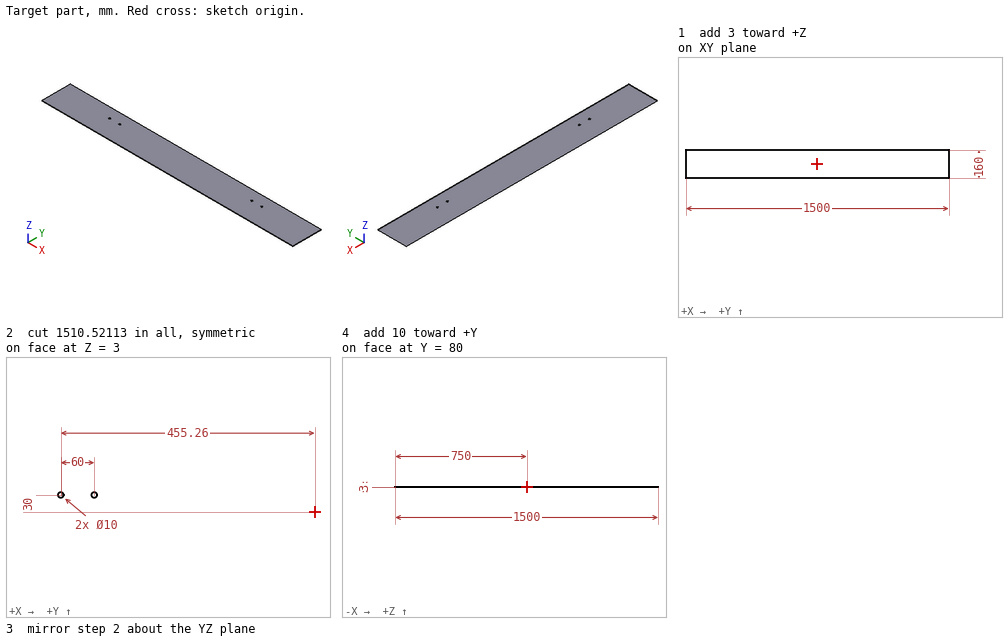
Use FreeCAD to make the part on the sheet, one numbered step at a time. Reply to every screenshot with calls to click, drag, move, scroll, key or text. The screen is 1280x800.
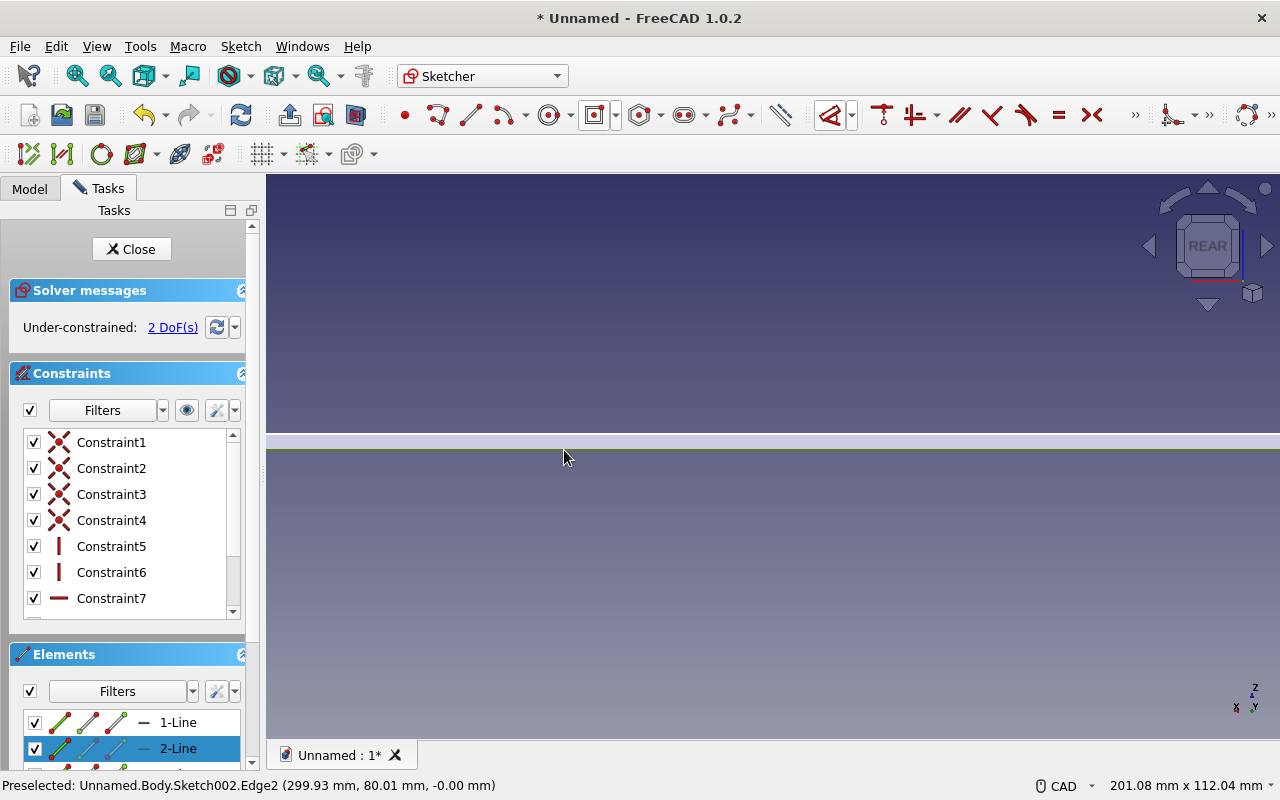
key(l)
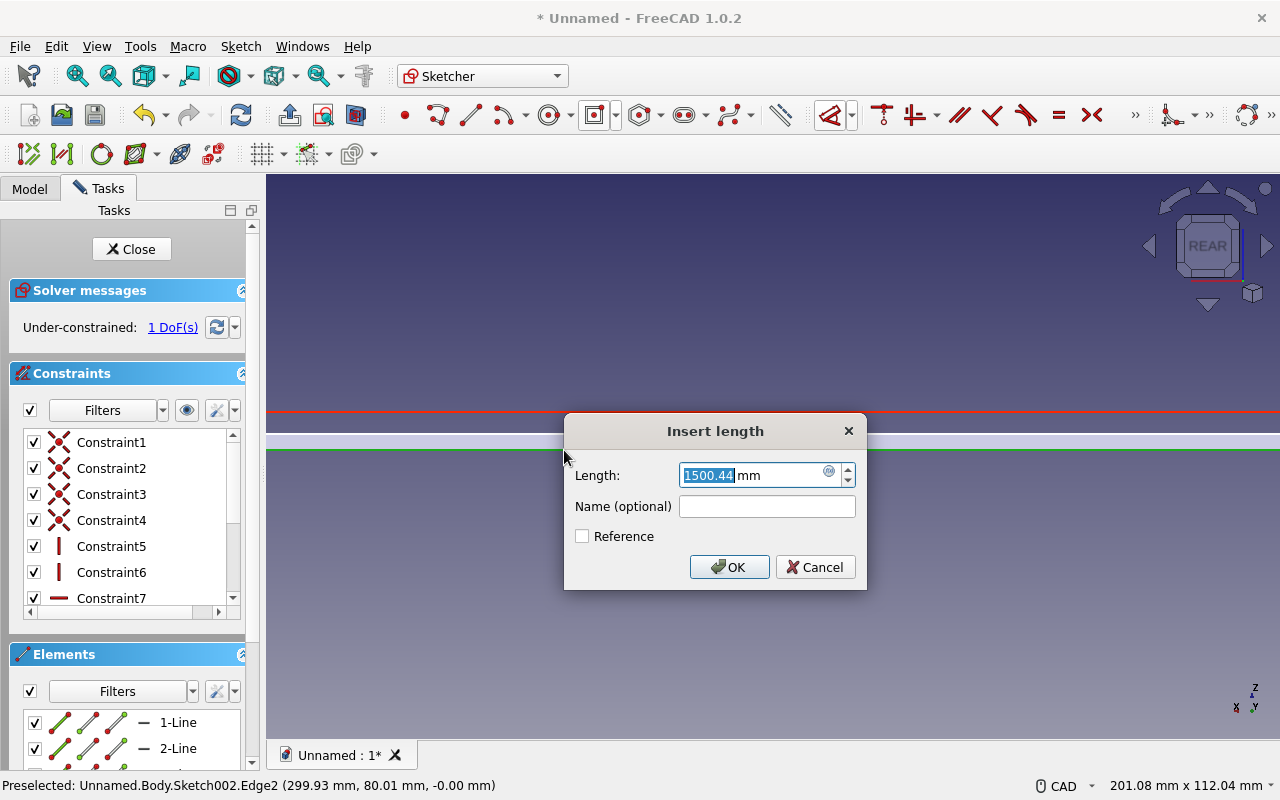
text(1500)
key(Return)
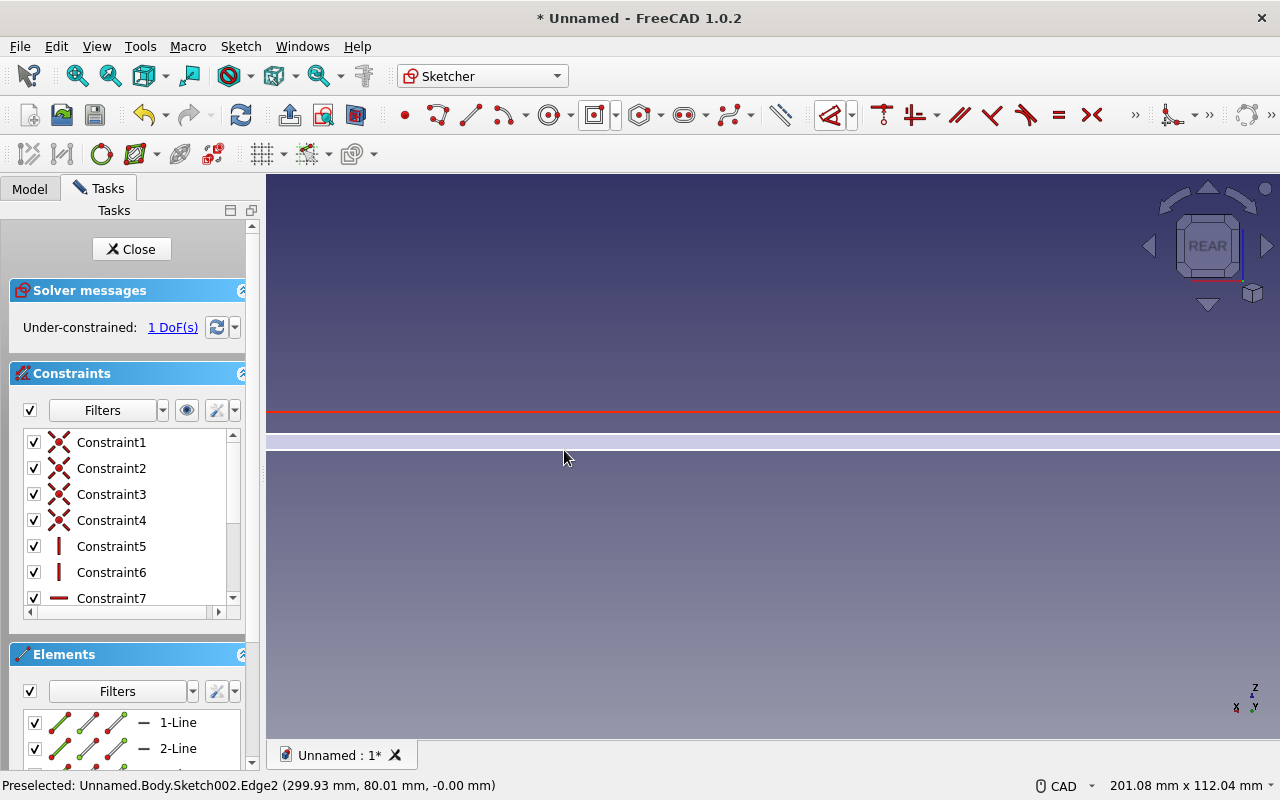
scroll(594, 458, down, 13)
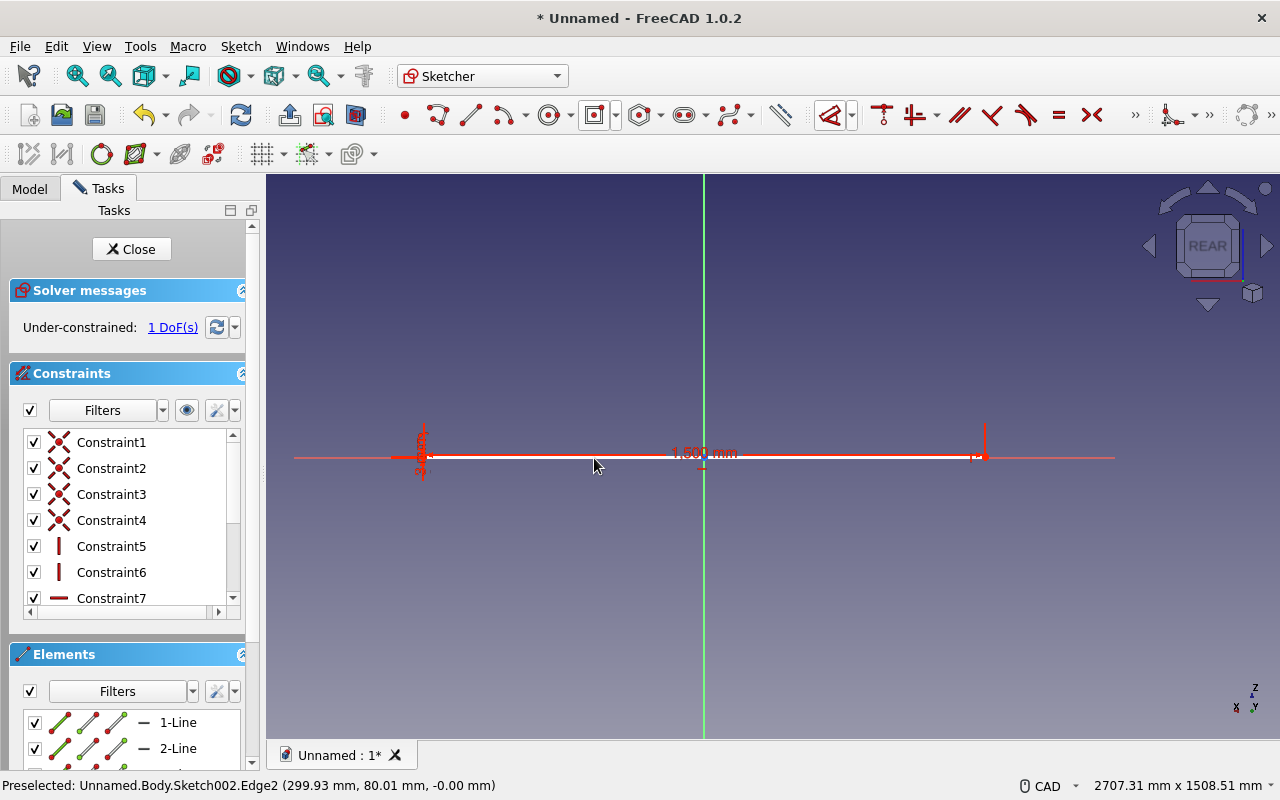
scroll(424, 457, up, 12)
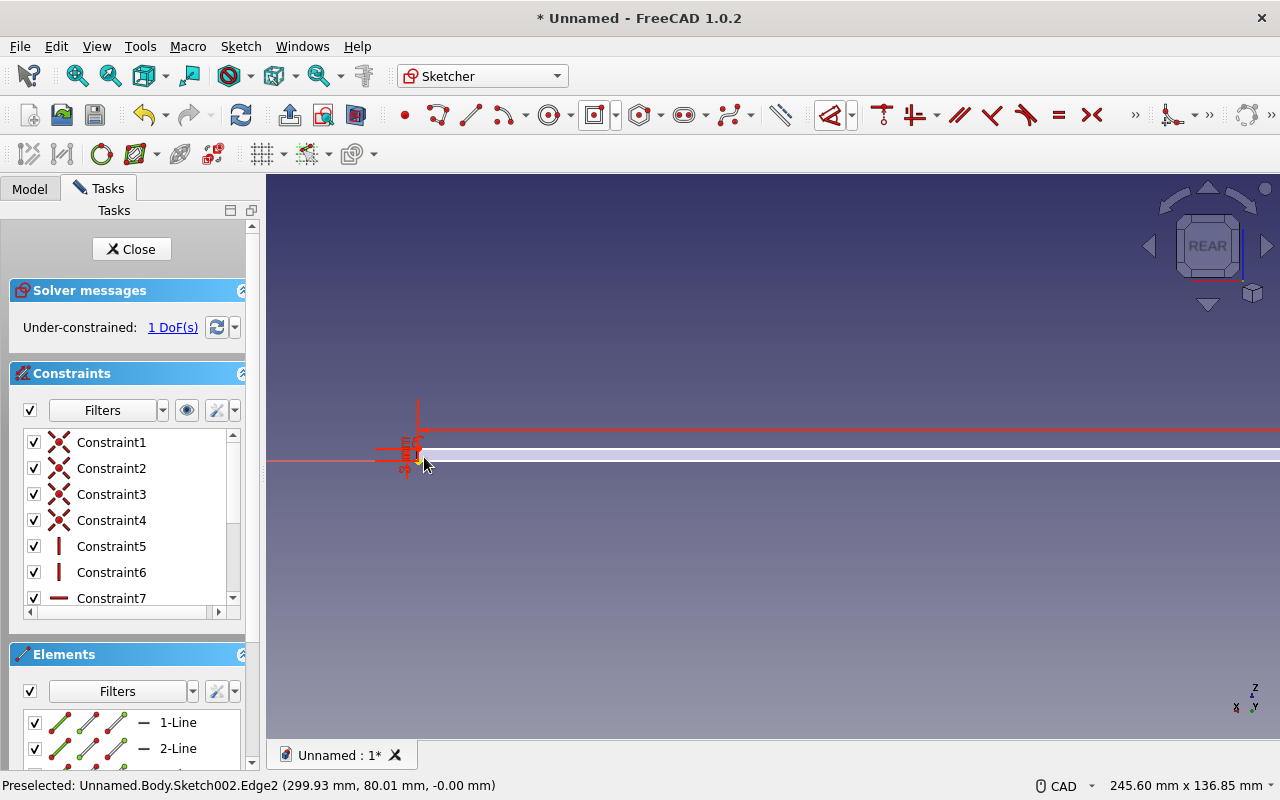
click(418, 449)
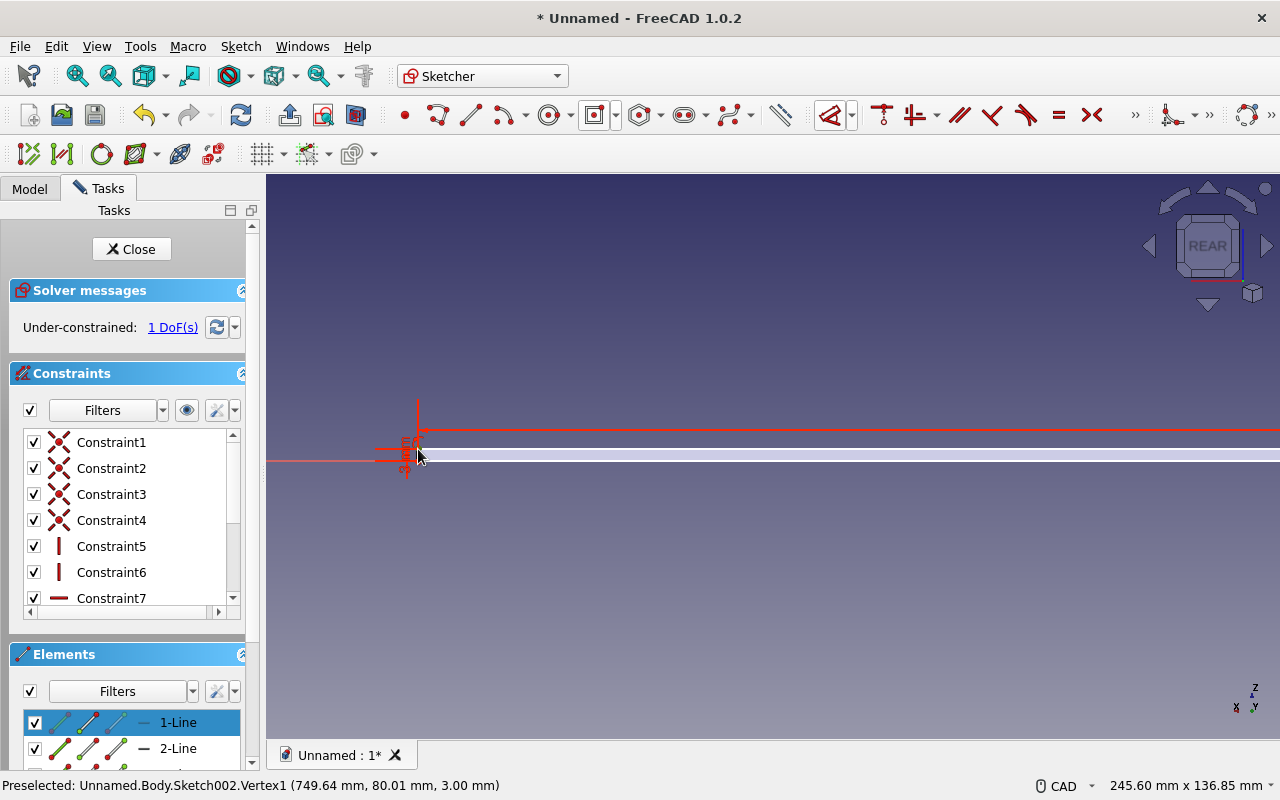
click(852, 116)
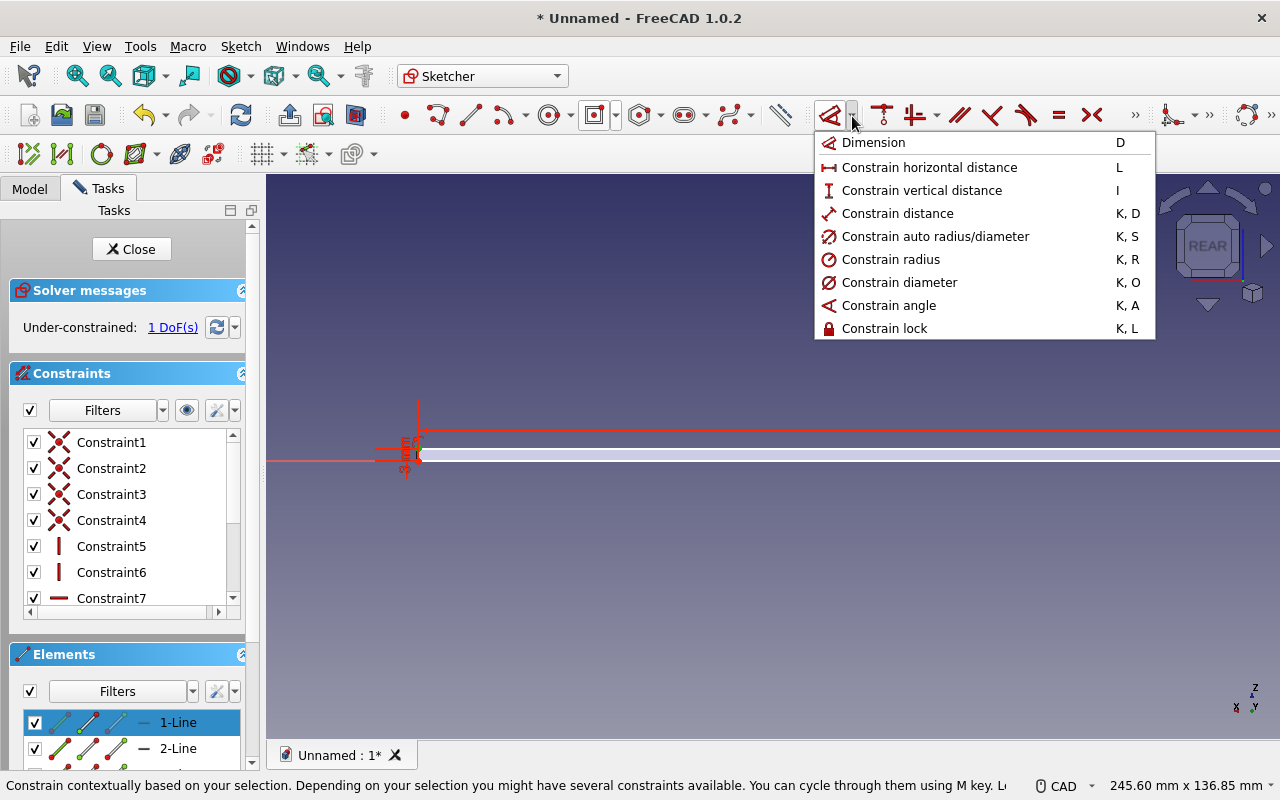
click(985, 168)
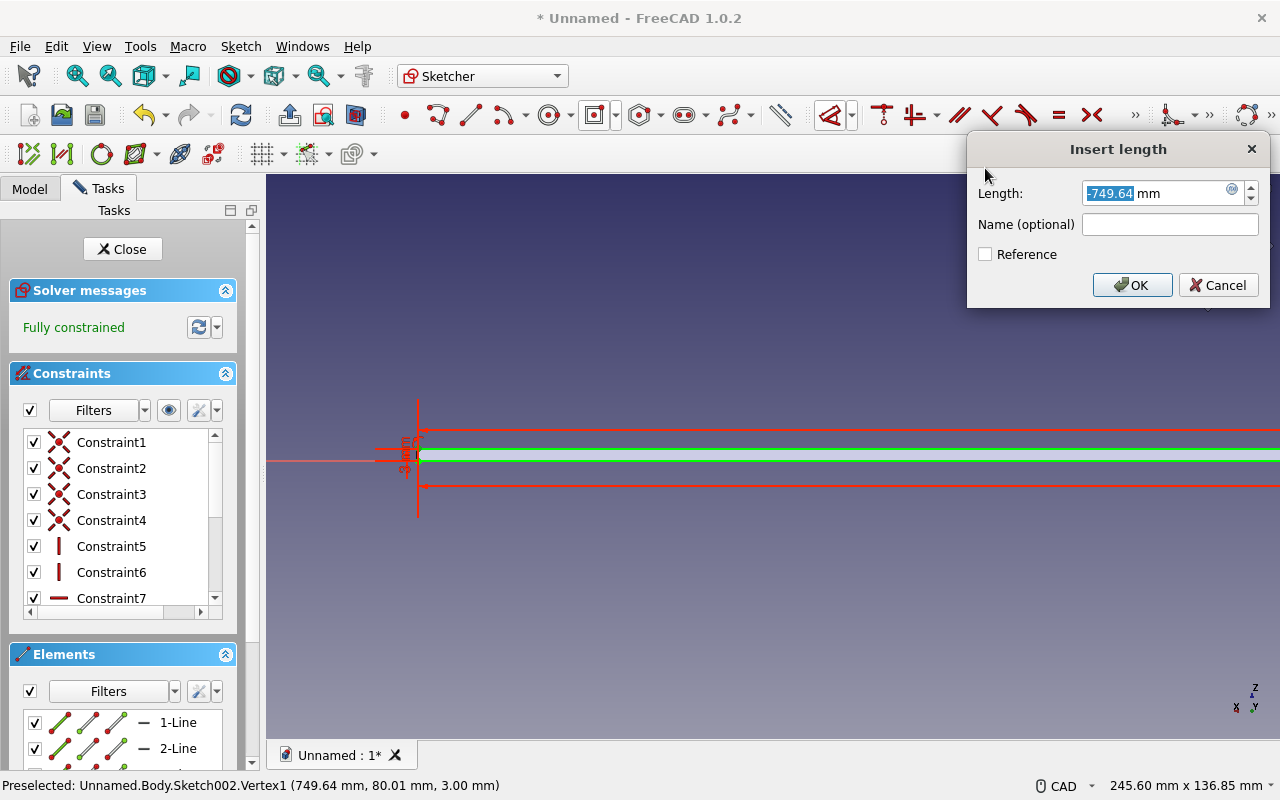
text(-750)
key(Return)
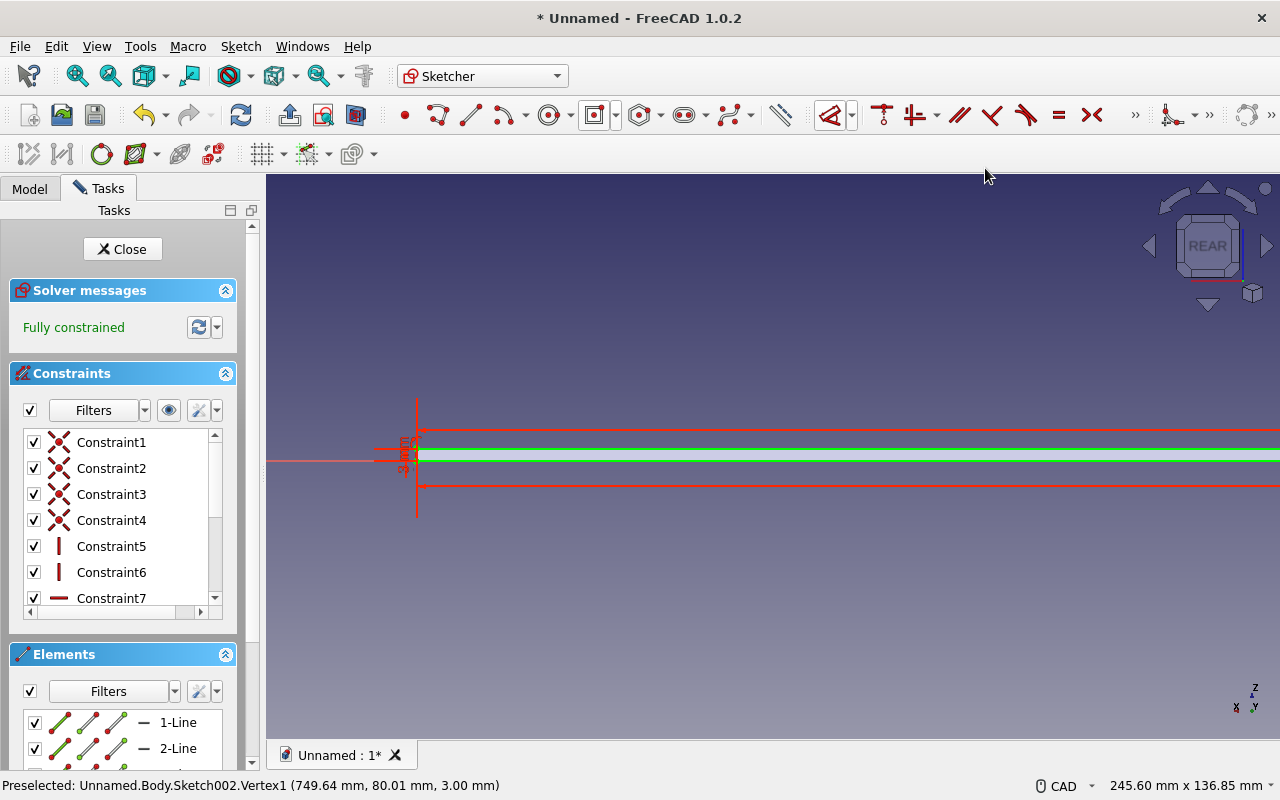
click(123, 249)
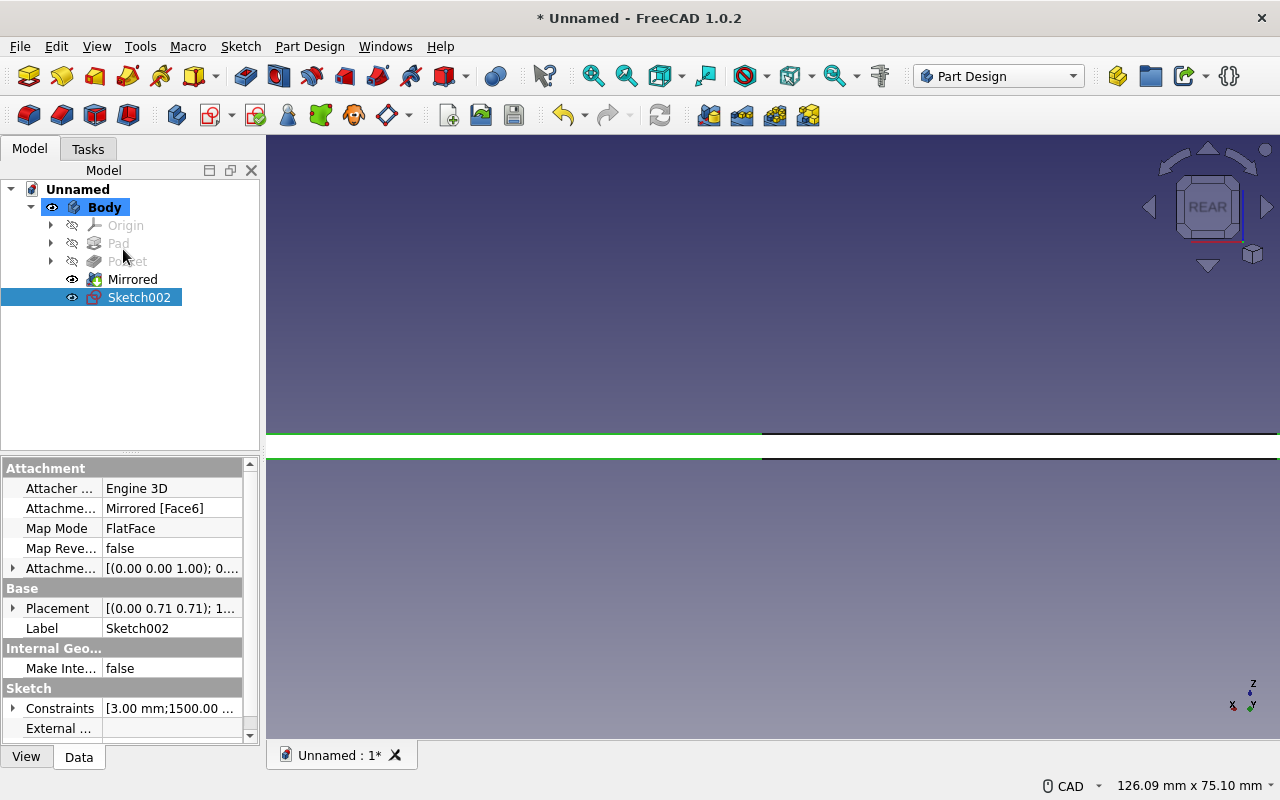
click(29, 76)